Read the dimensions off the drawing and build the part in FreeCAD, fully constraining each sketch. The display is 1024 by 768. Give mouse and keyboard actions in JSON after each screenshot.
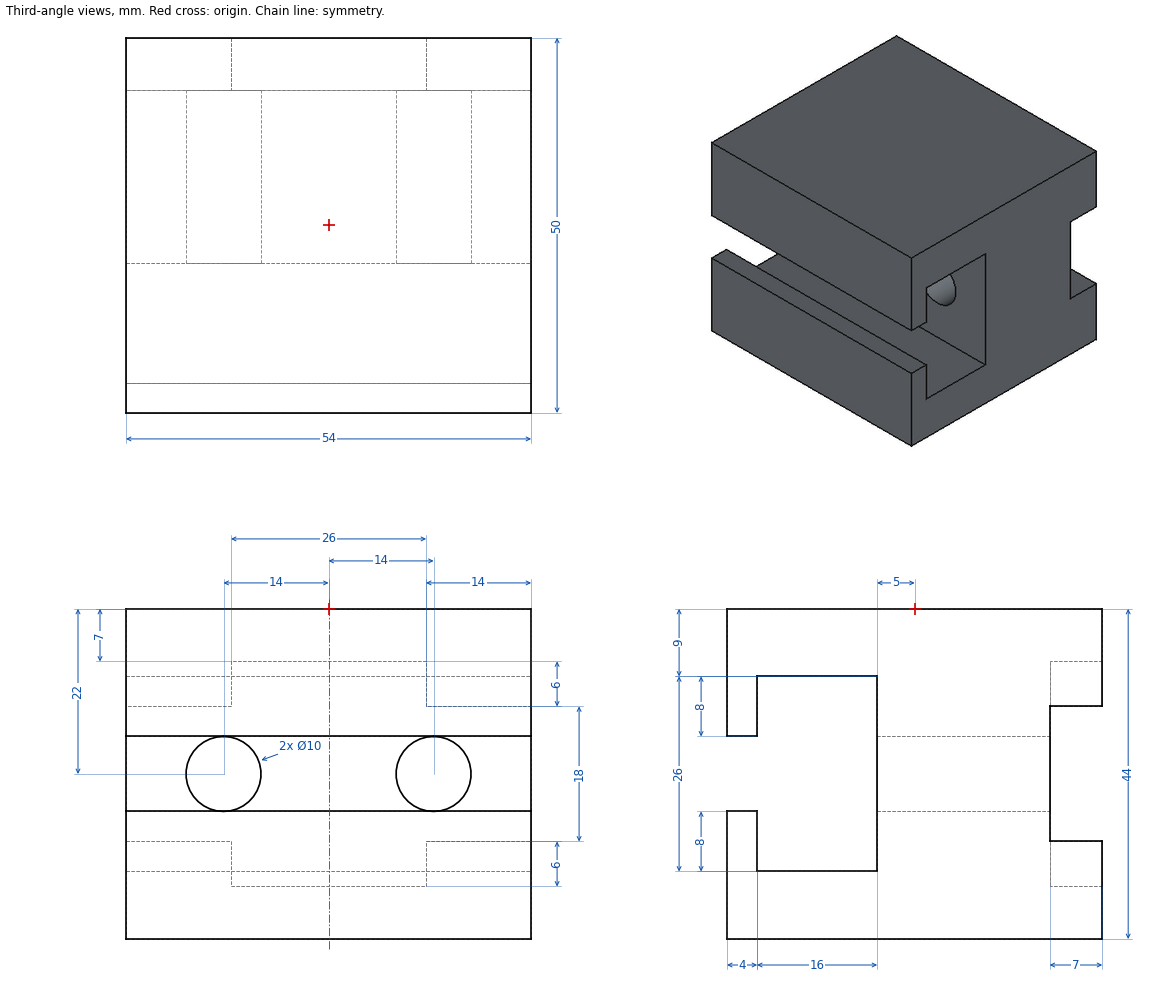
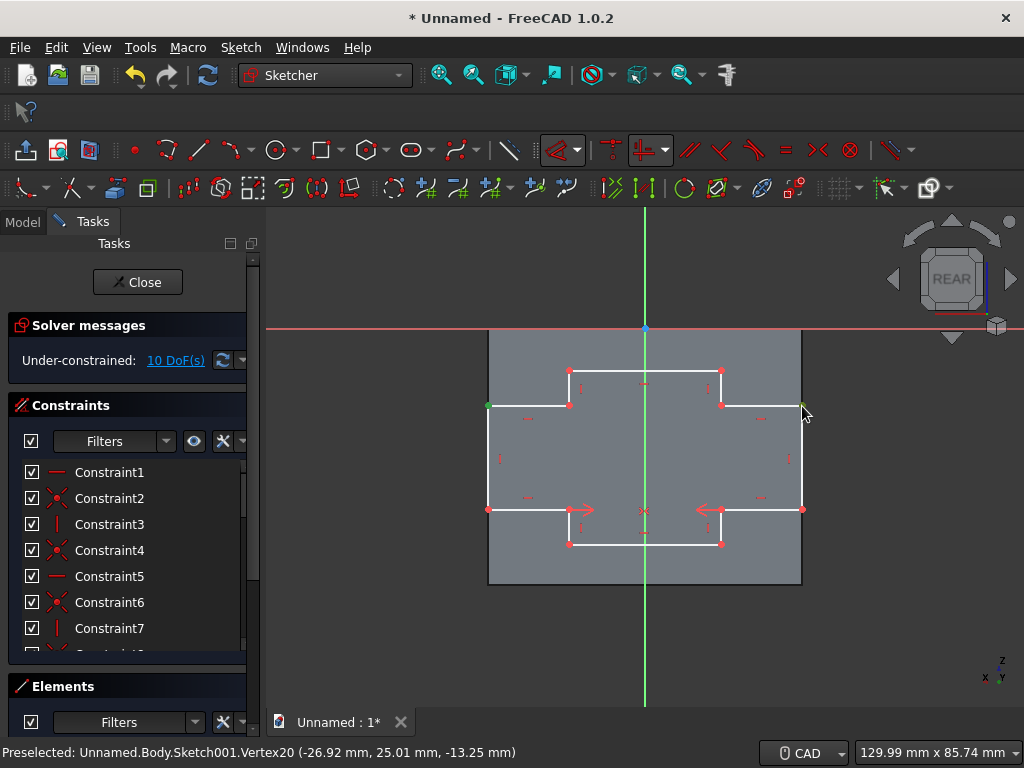
{"action": "left_click", "coordinate": [645, 647]}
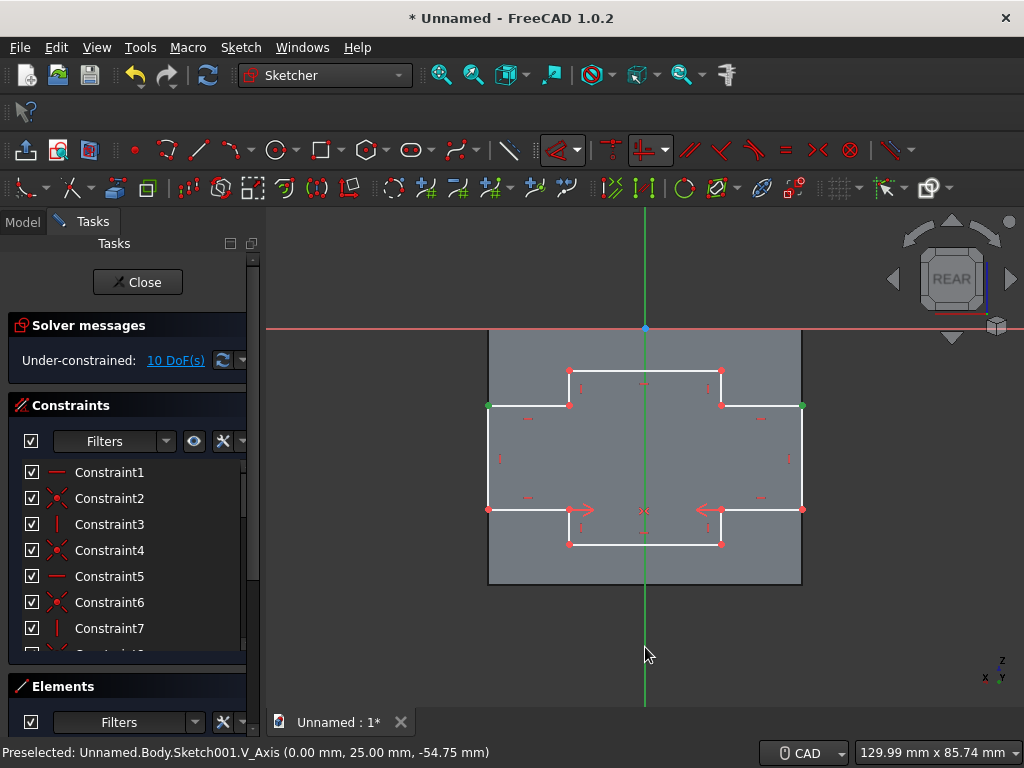
{"action": "key", "text": "s"}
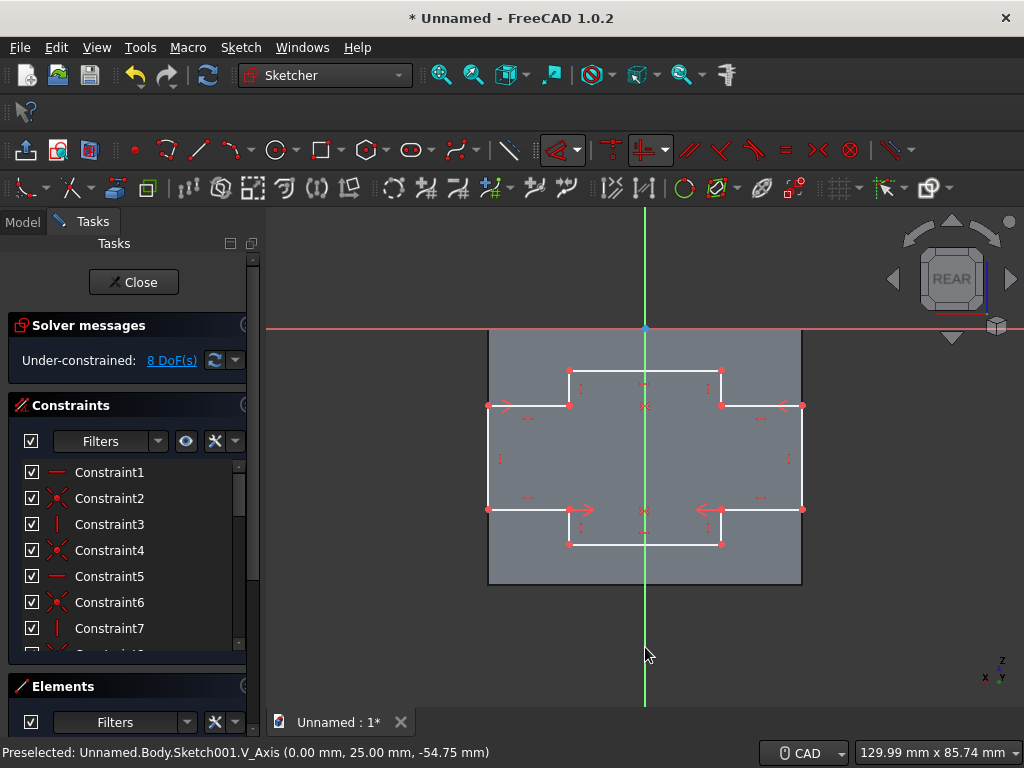
{"action": "left_click", "coordinate": [556, 150]}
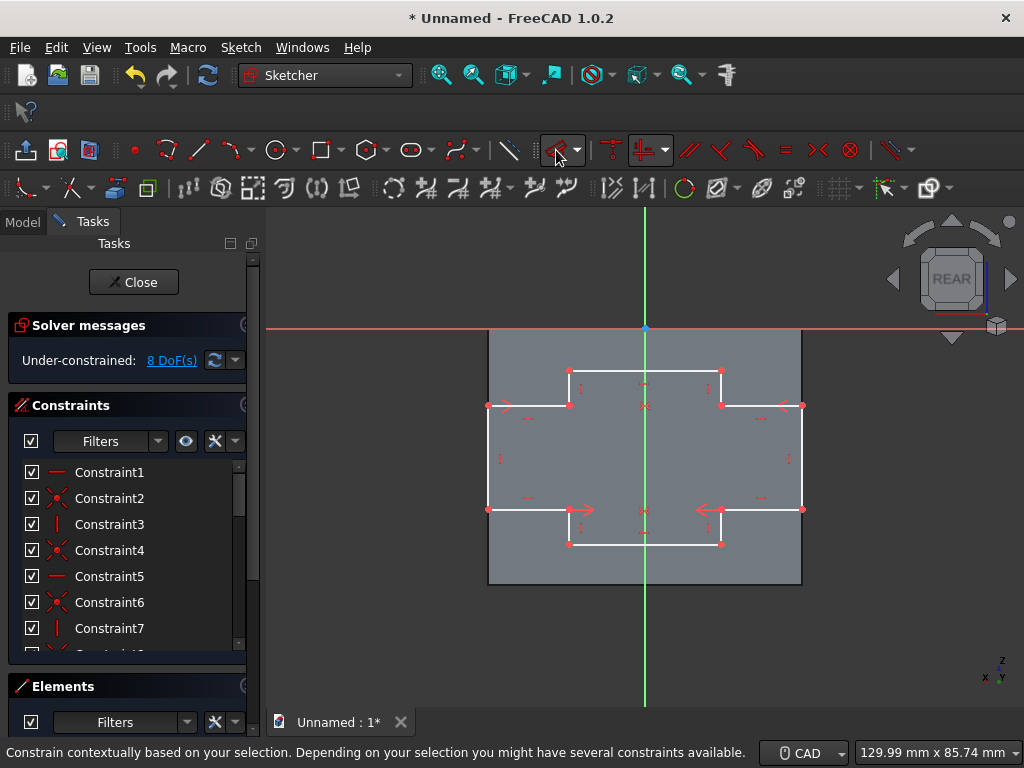
{"action": "scroll", "coordinate": [569, 382], "scroll_direction": "up", "scroll_amount": 2}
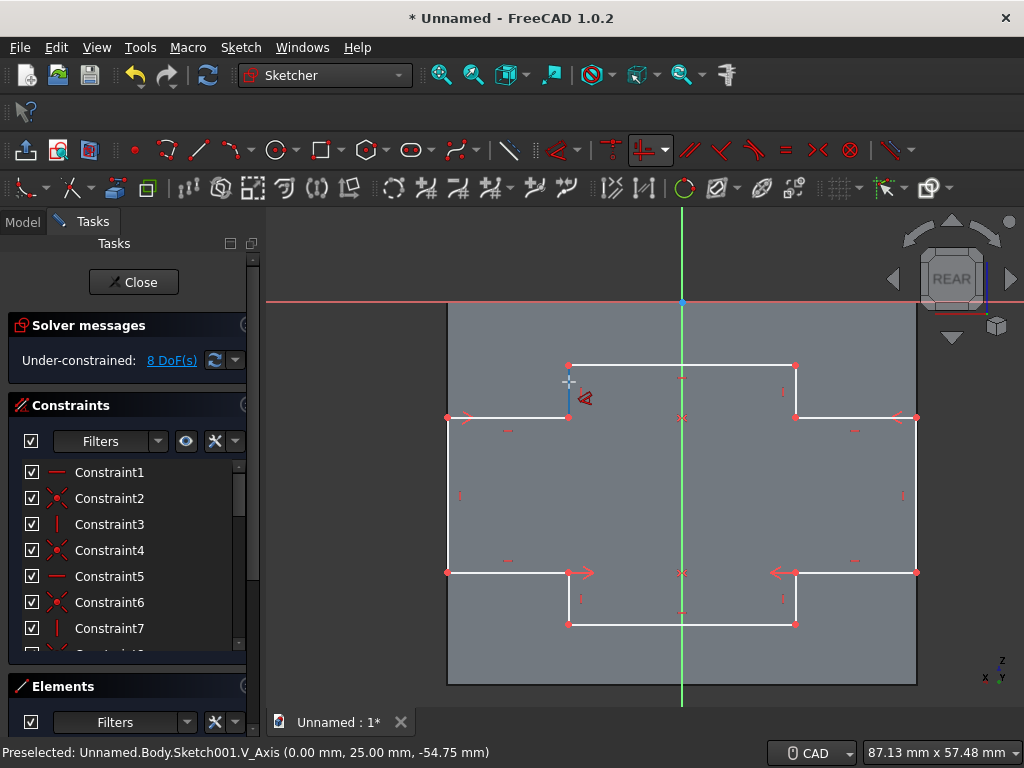
{"action": "left_click", "coordinate": [569, 381]}
{"action": "left_click", "coordinate": [535, 392]}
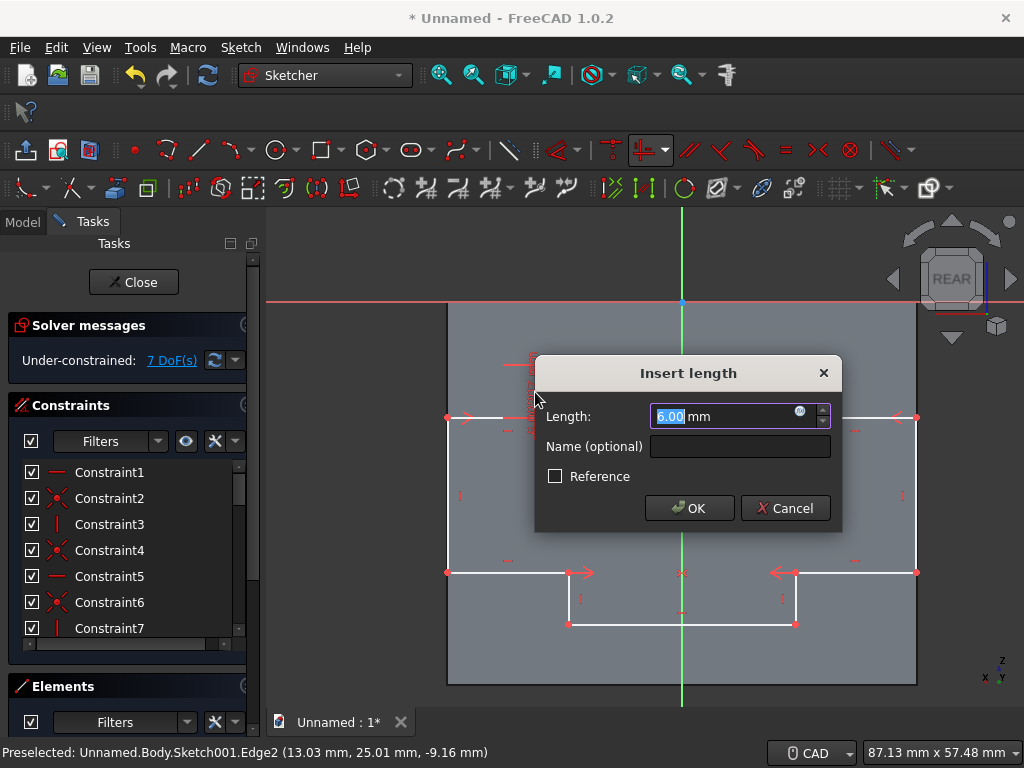
{"action": "type", "text": "6"}
{"action": "key", "text": "Return"}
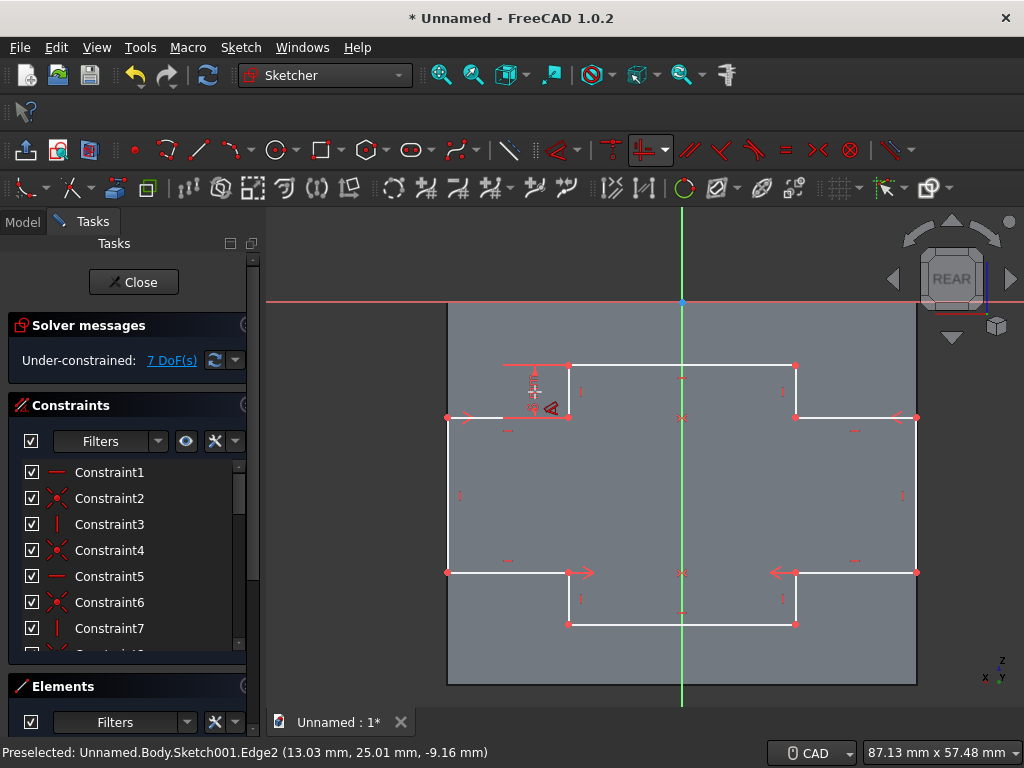
{"action": "left_click", "coordinate": [569, 588]}
{"action": "left_click", "coordinate": [535, 599]}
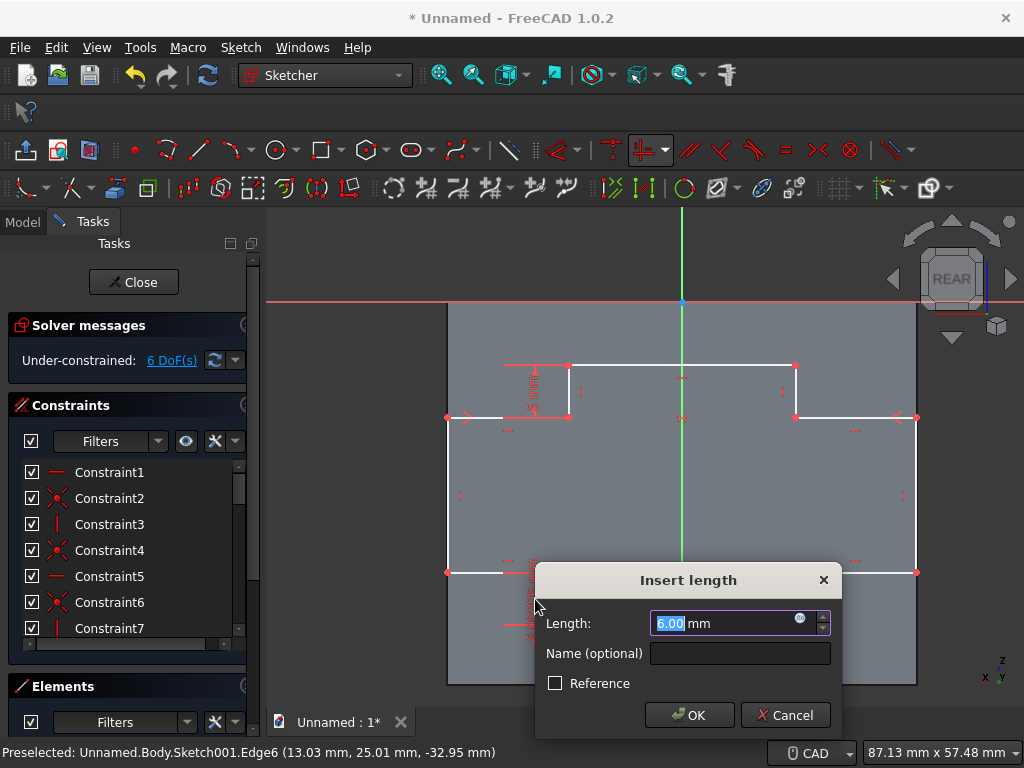
{"action": "type", "text": "6"}
{"action": "key", "text": "Return"}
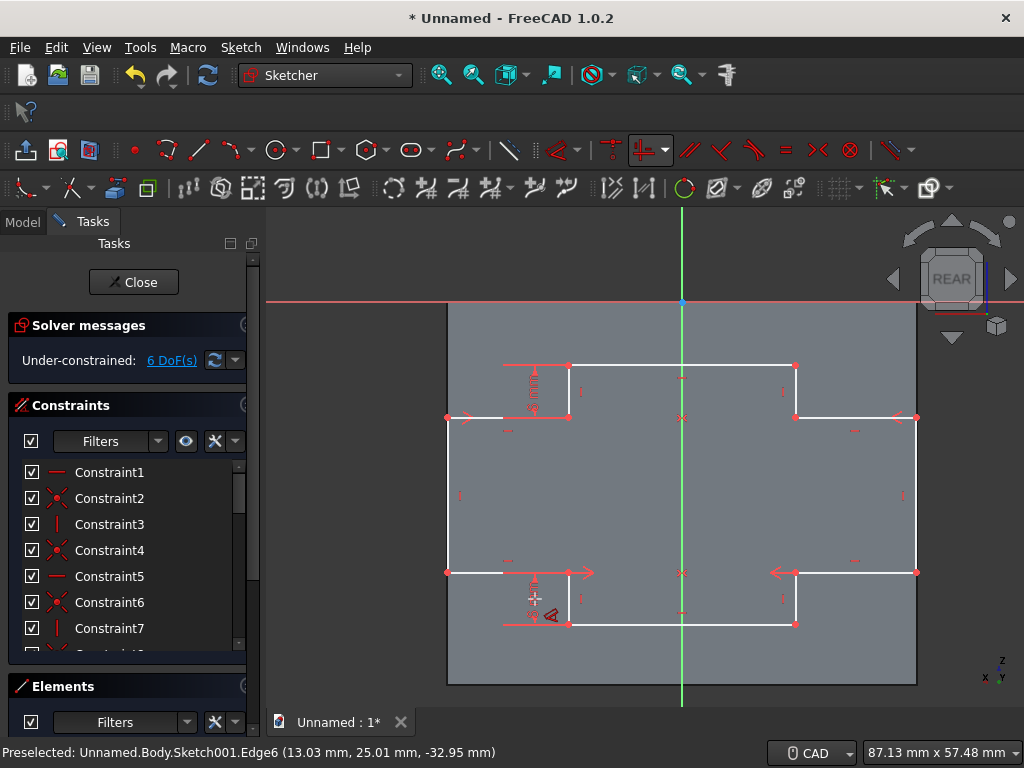
{"action": "left_click", "coordinate": [728, 365]}
{"action": "left_click", "coordinate": [630, 331]}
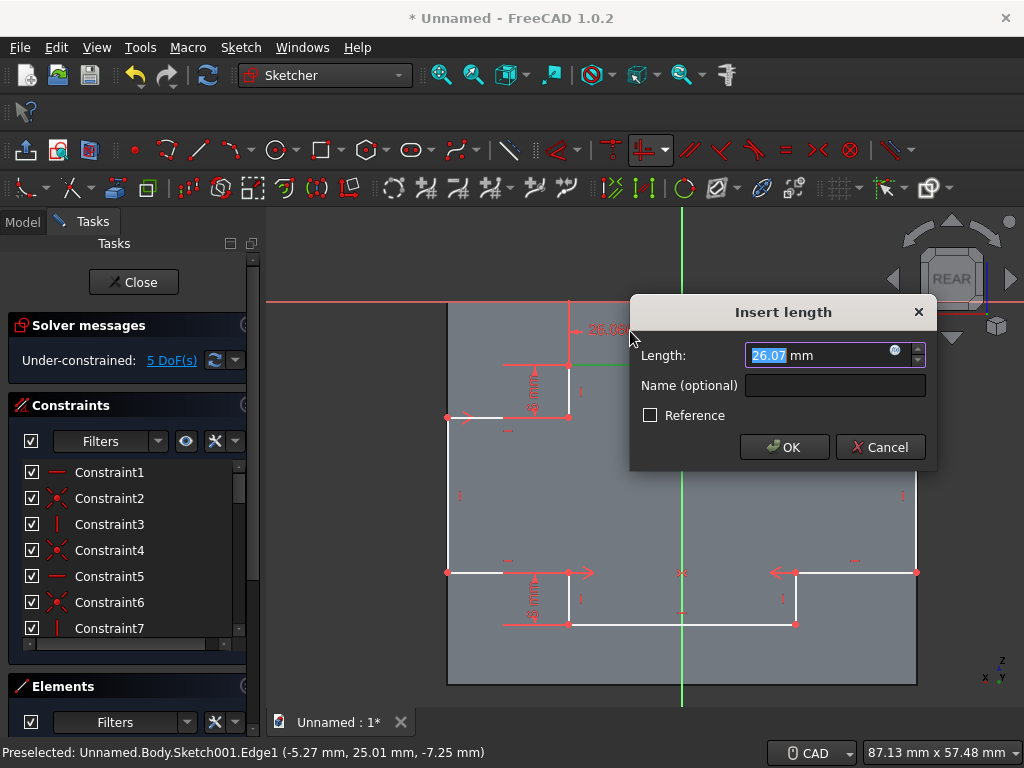
{"action": "type", "text": "26"}
{"action": "key", "text": "Return"}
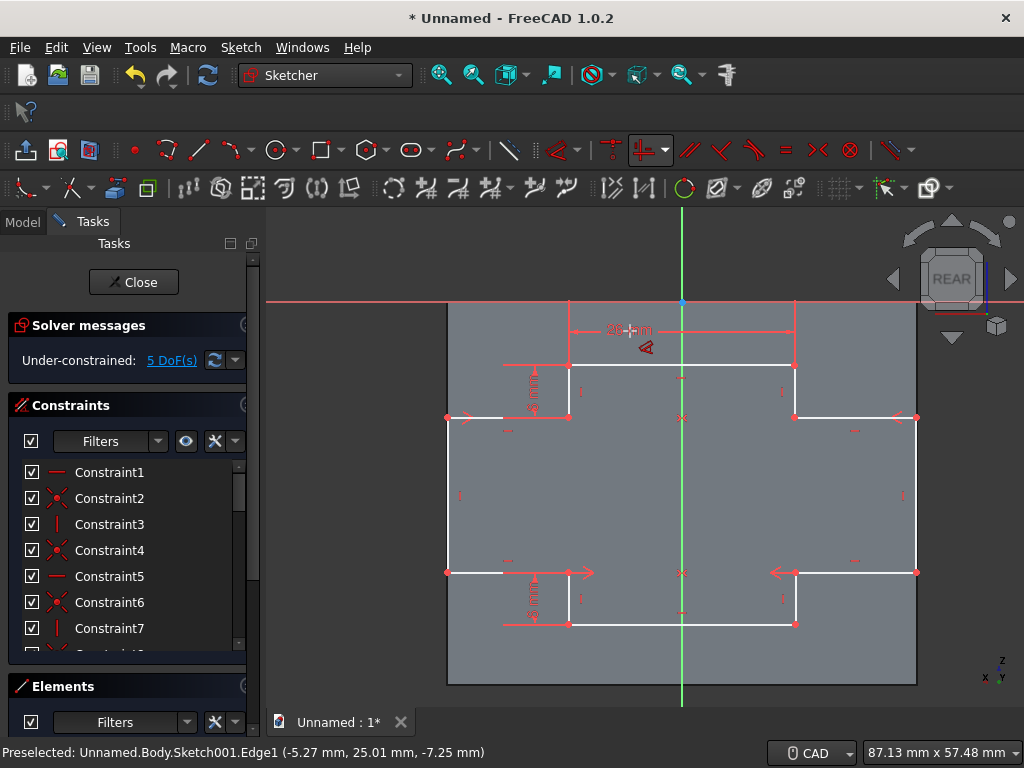
{"action": "left_click", "coordinate": [533, 418]}
{"action": "left_click", "coordinate": [508, 452]}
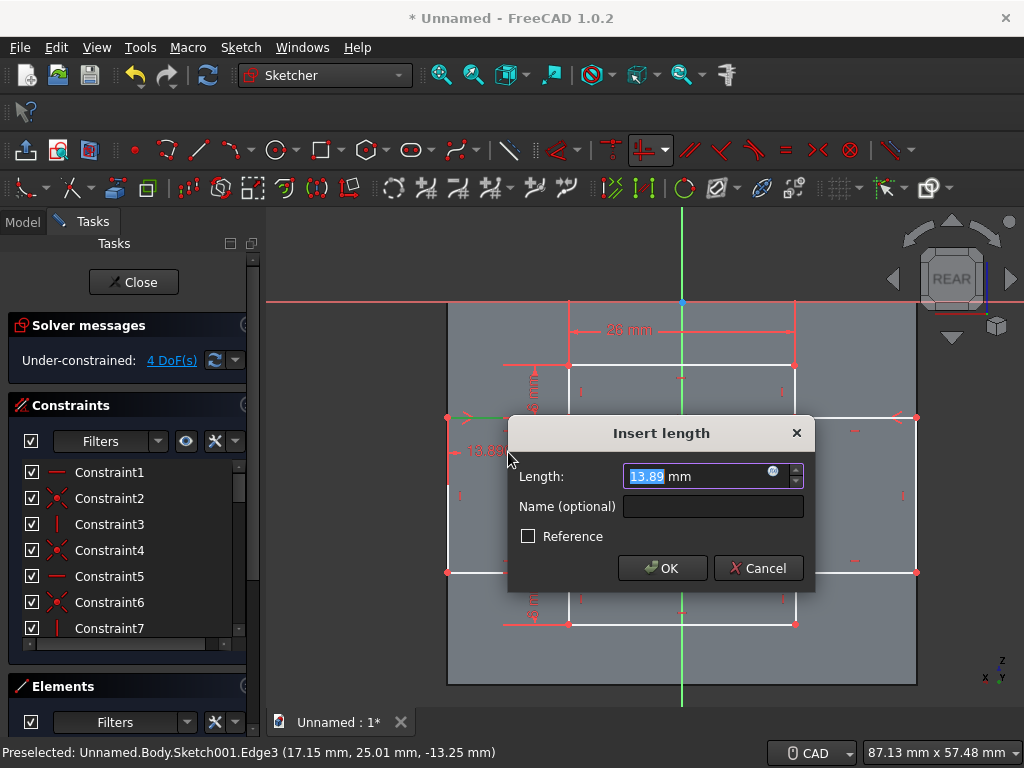
{"action": "type", "text": "14"}
{"action": "key", "text": "Return"}